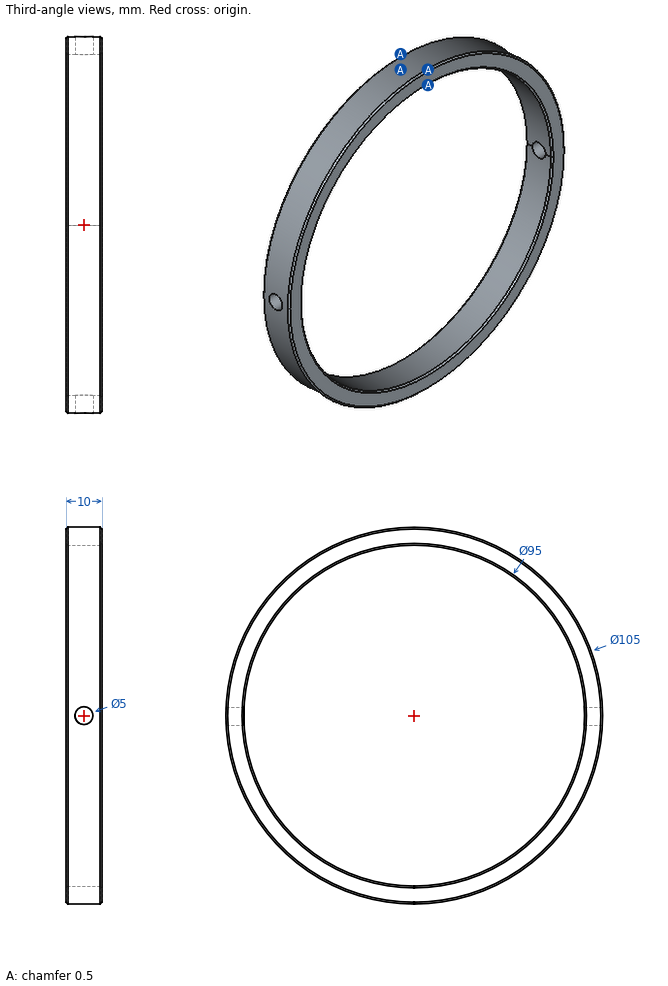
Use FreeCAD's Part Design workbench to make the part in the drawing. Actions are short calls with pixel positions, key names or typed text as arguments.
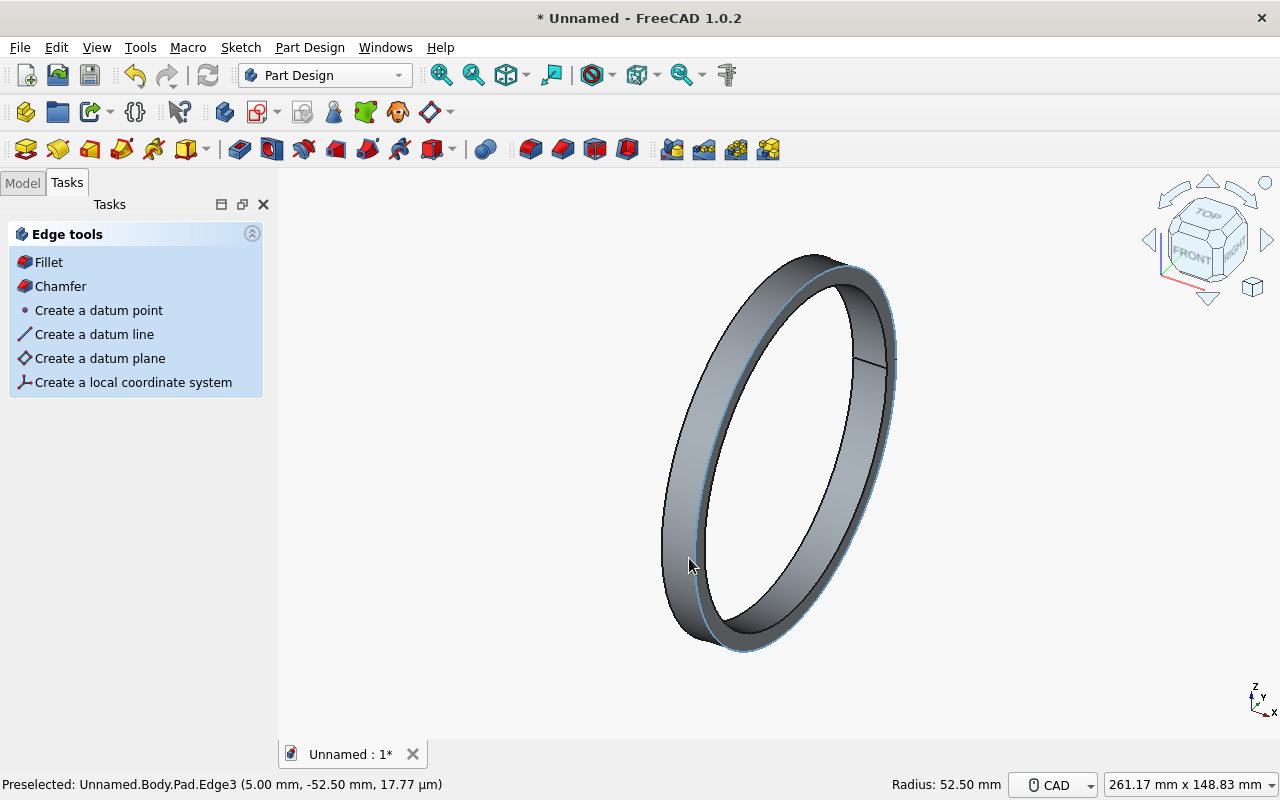
click(767, 628, ctrl)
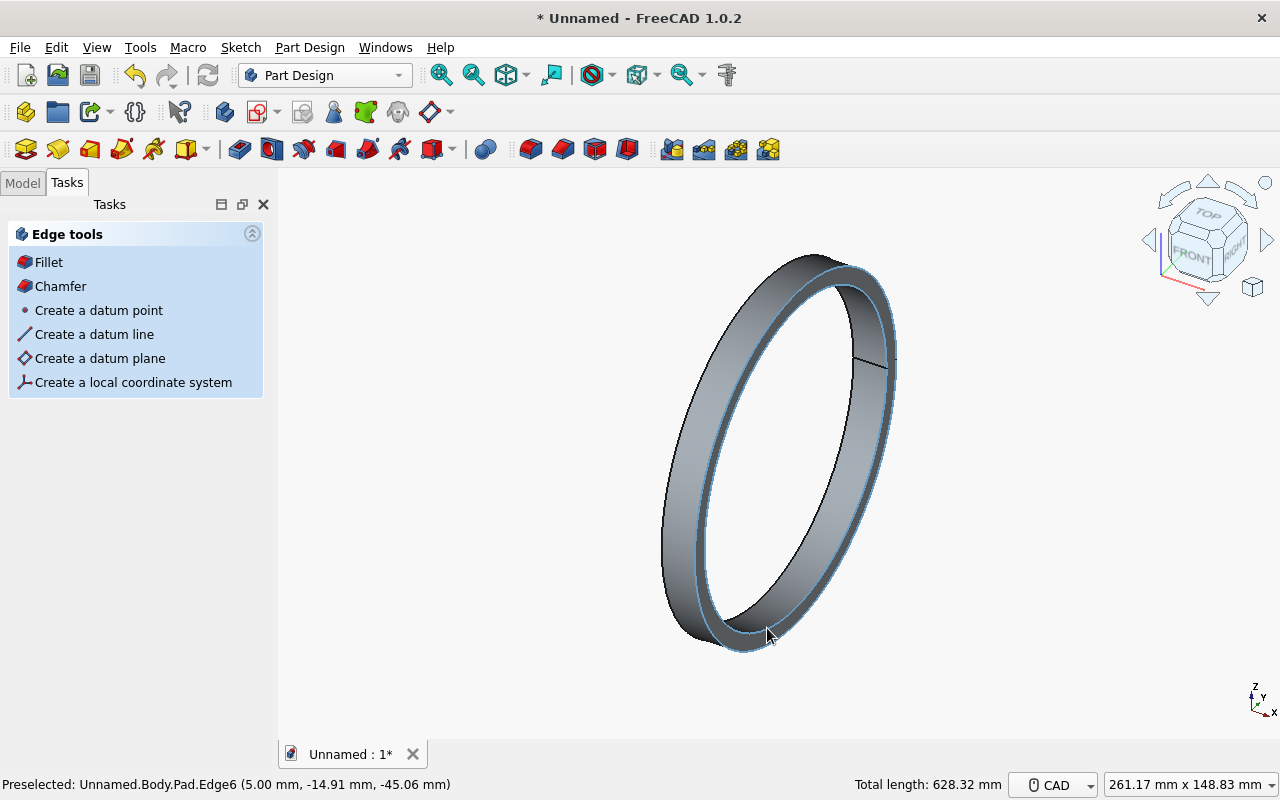
key(0)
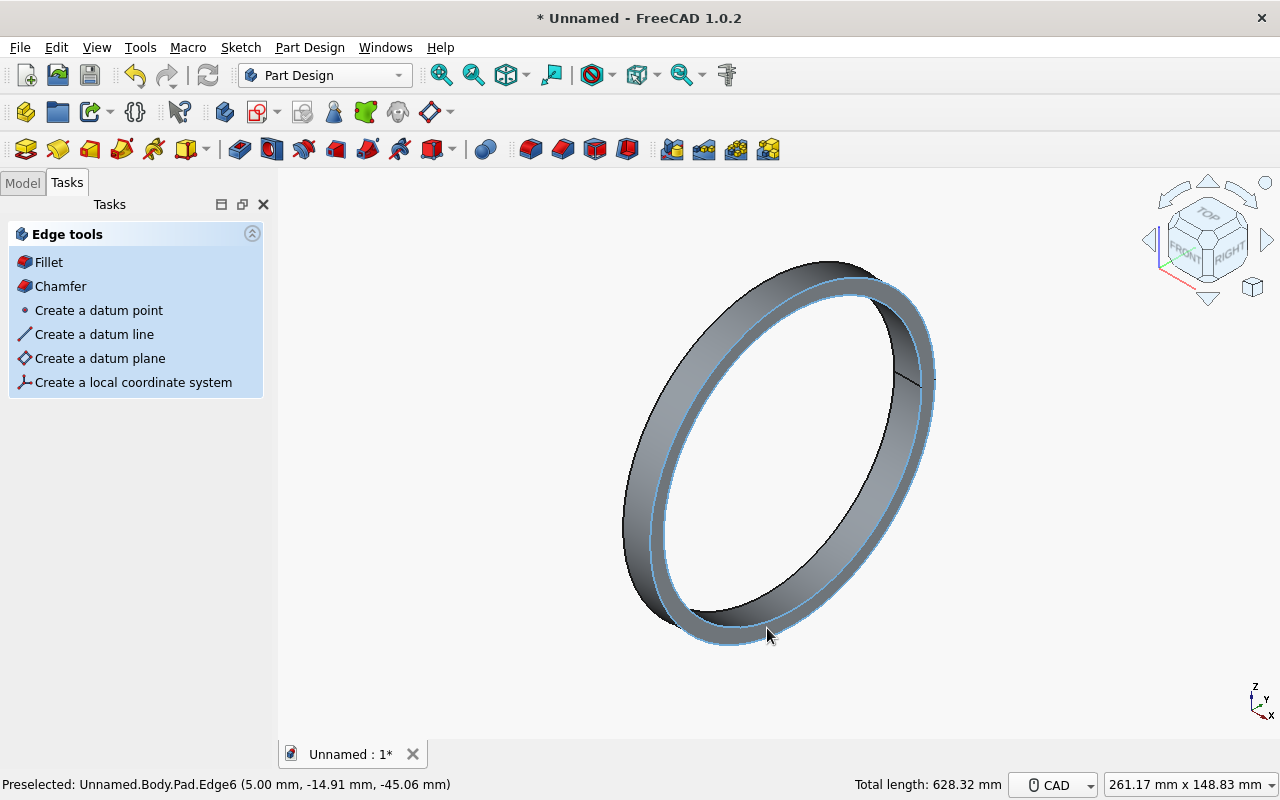
key(2)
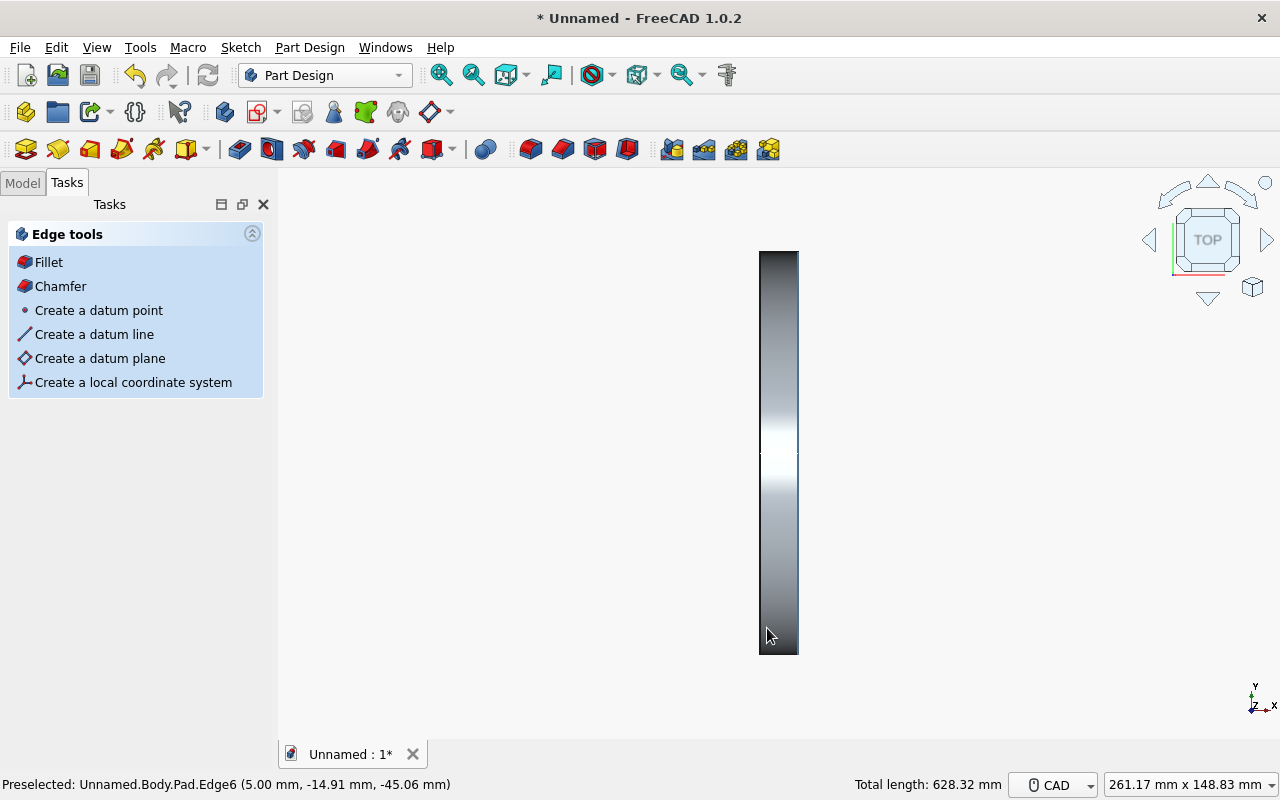
click(760, 615, ctrl)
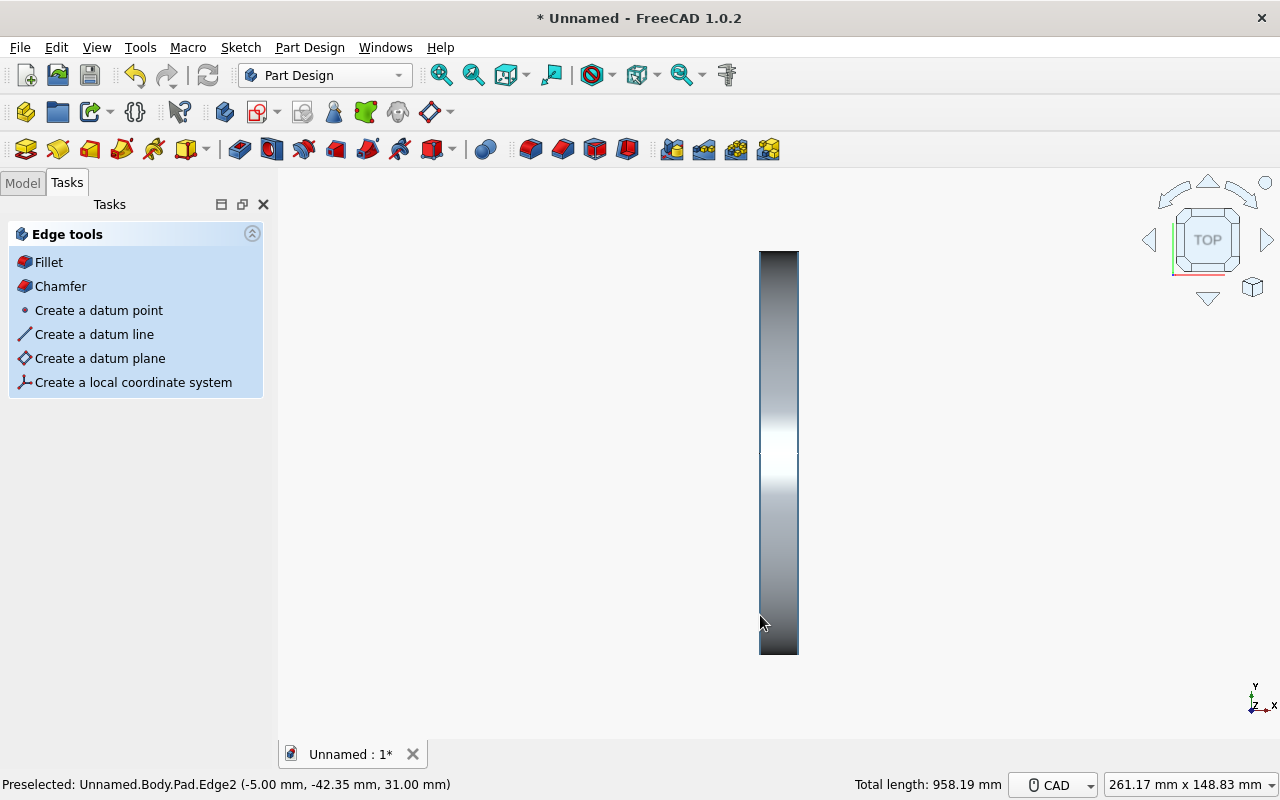
key(1)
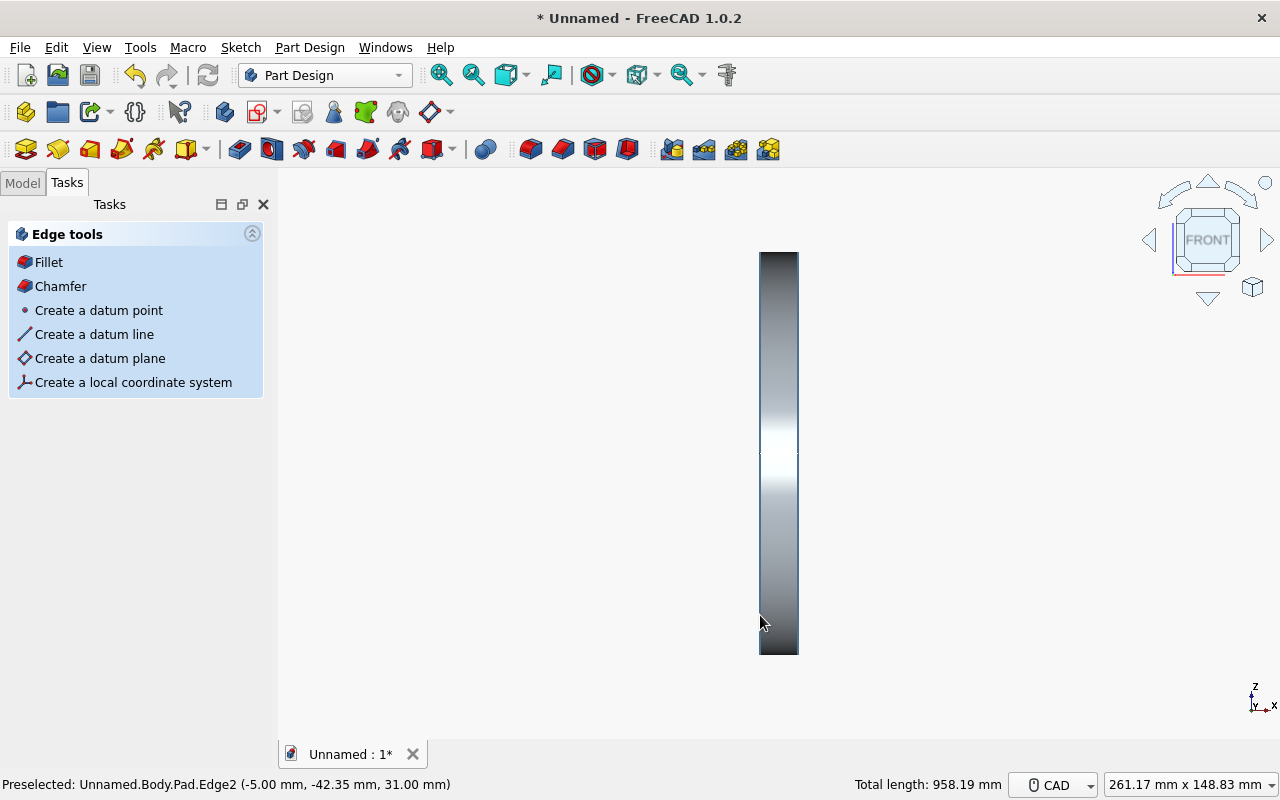
key(3)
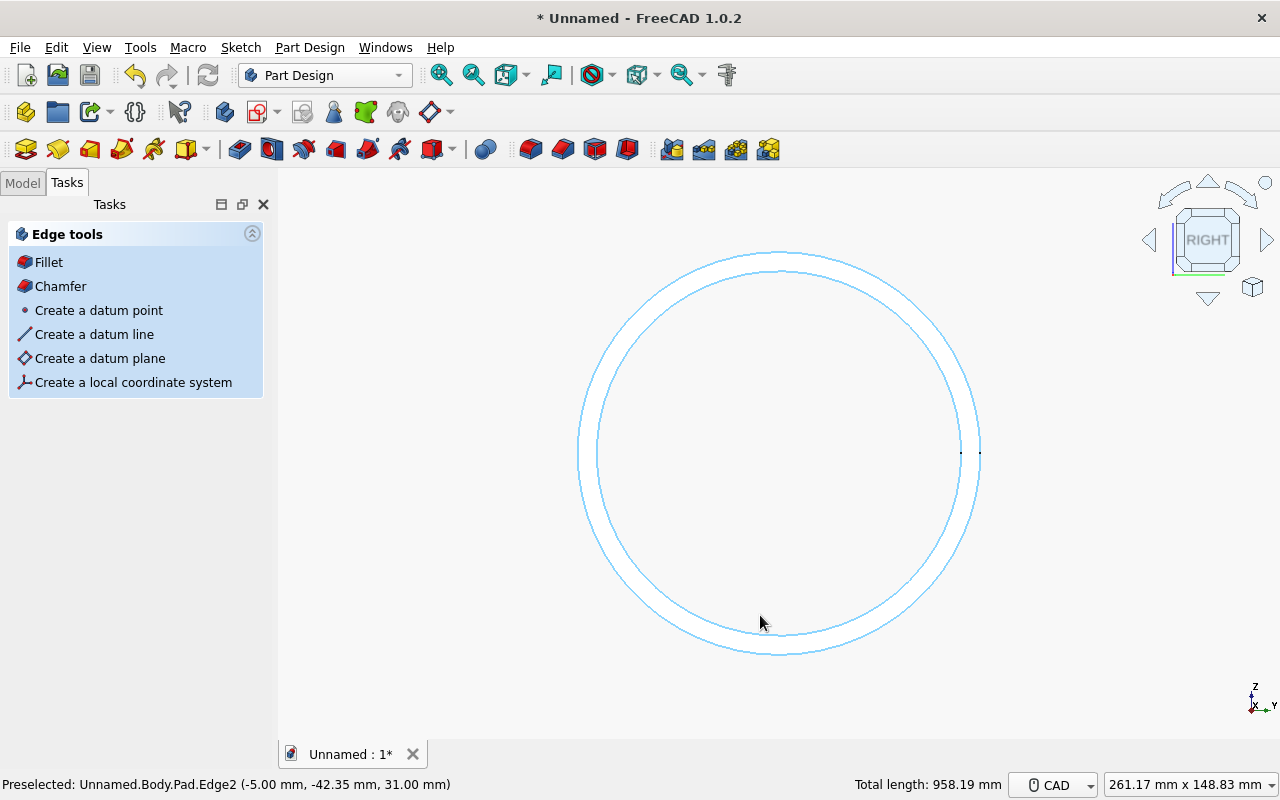
key(5)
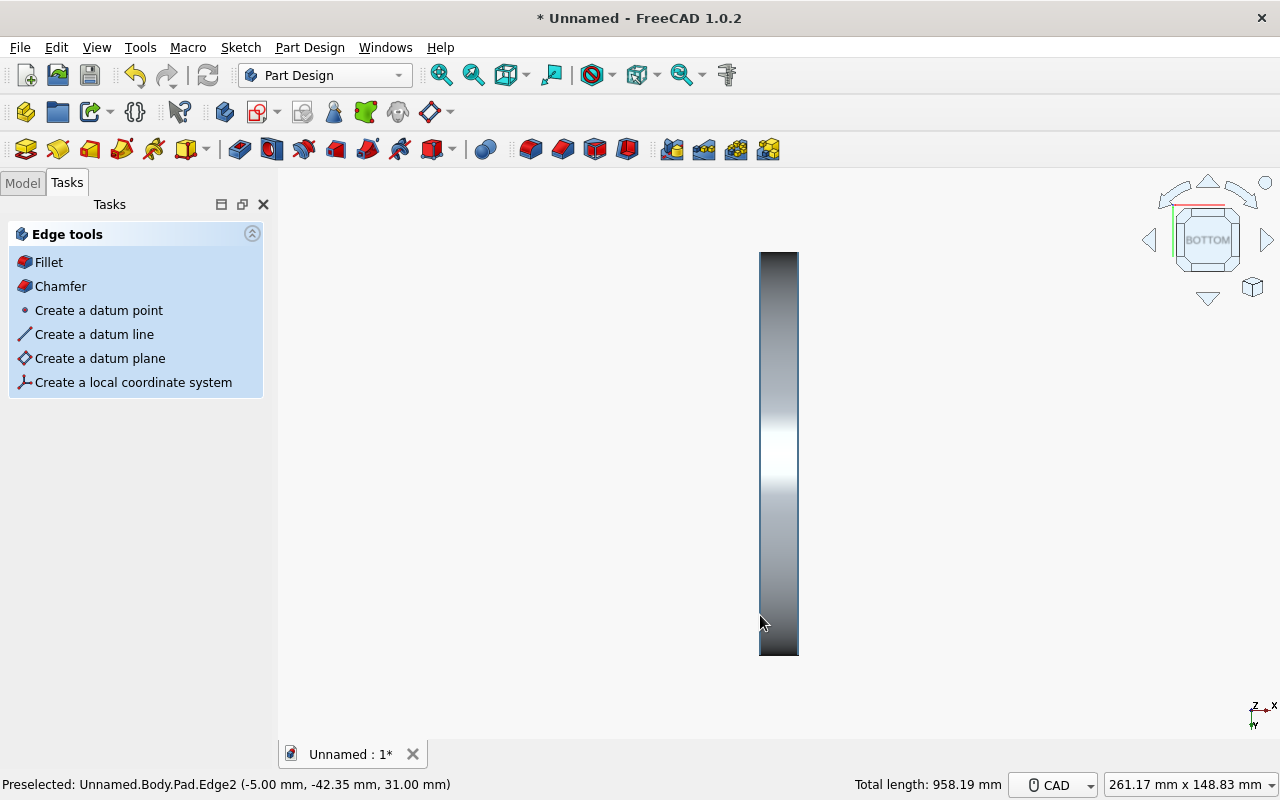
key(4)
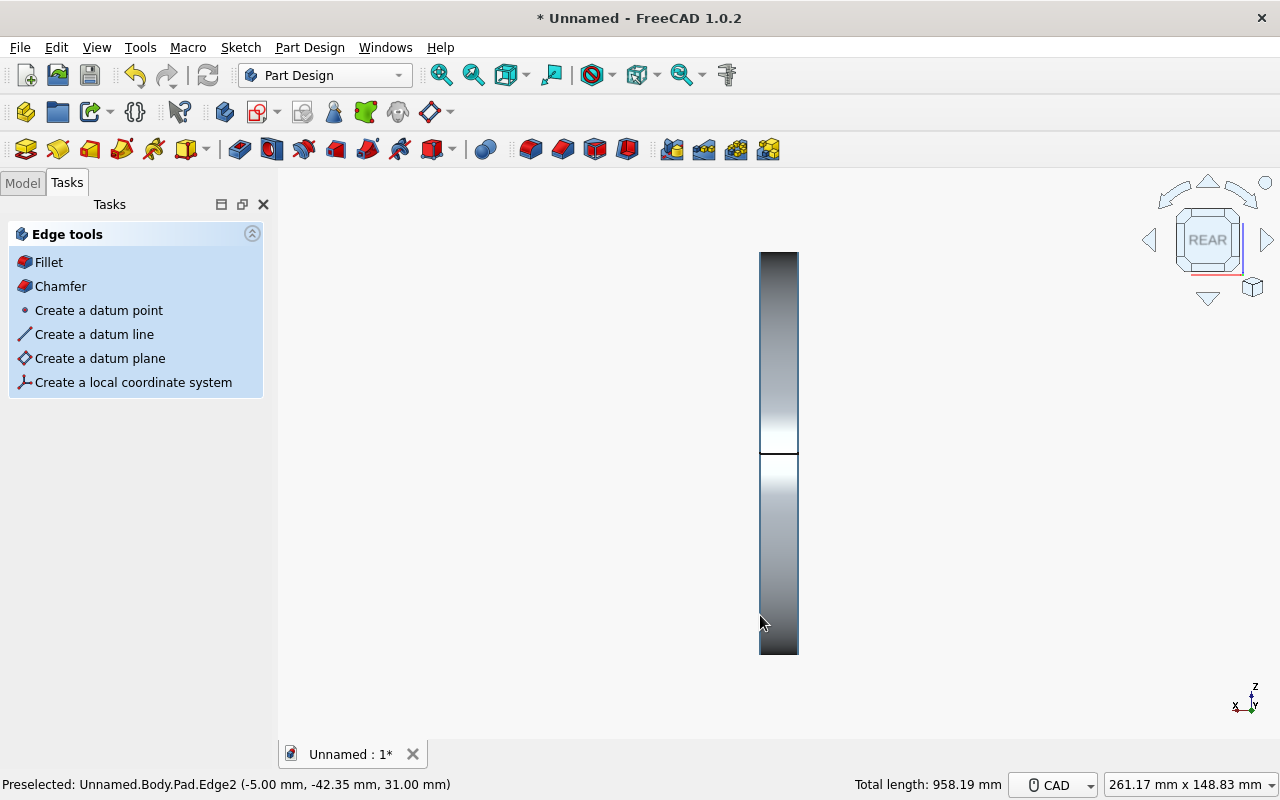
key(6)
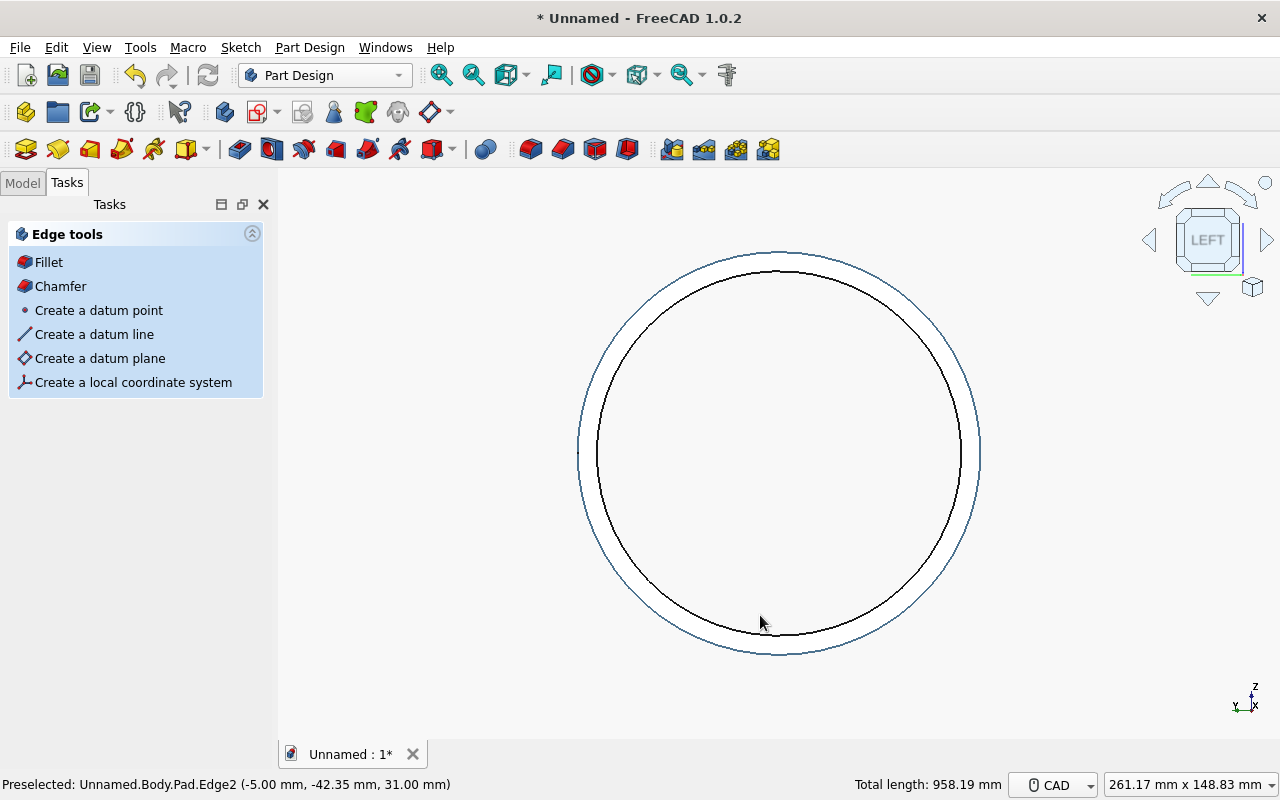
click(961, 452, ctrl)